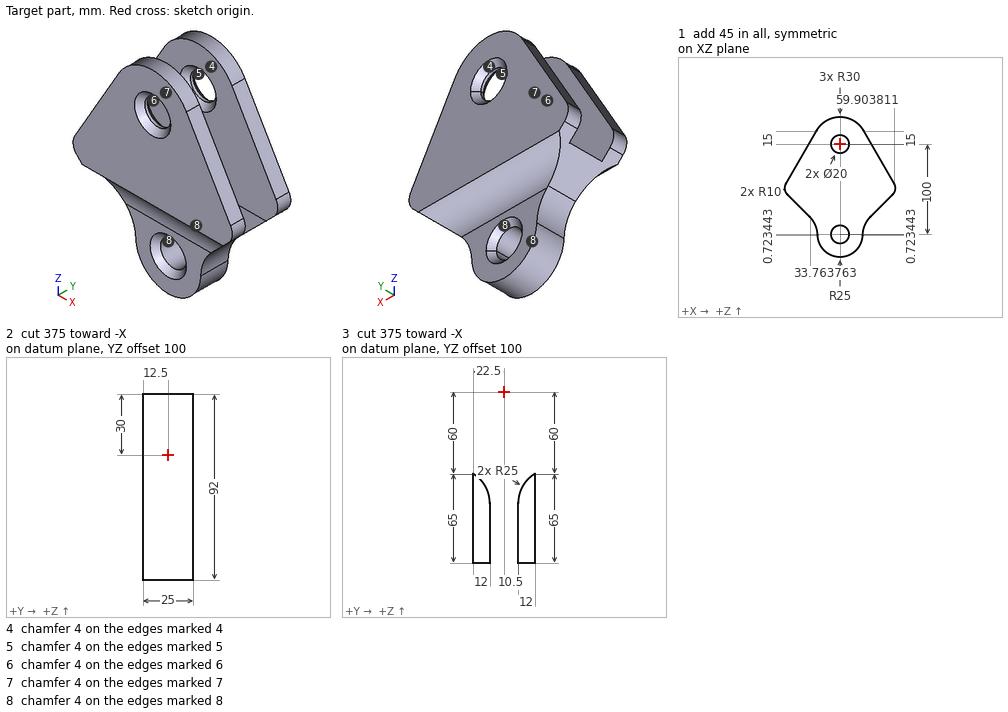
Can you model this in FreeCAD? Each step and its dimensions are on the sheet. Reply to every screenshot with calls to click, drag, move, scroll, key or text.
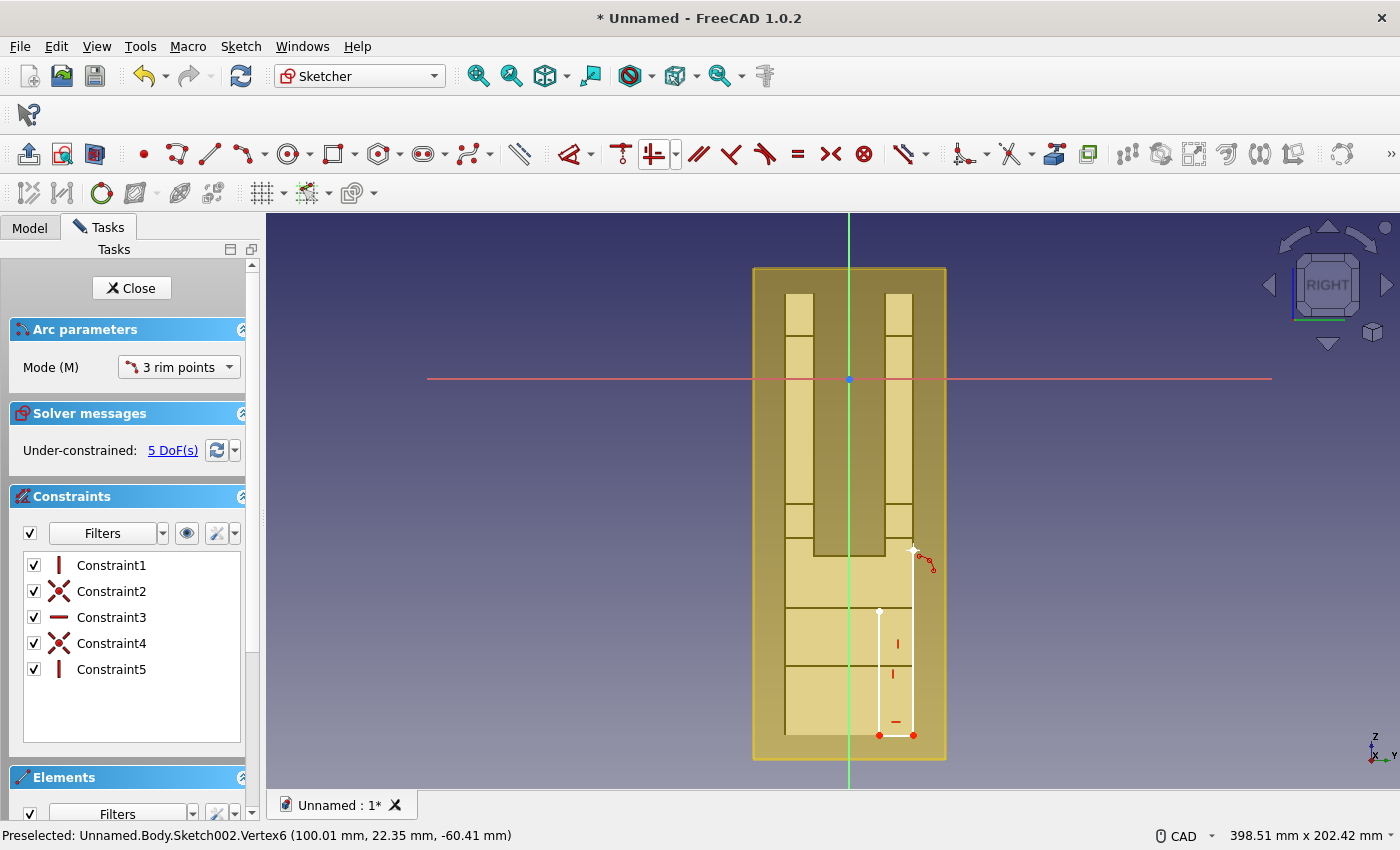
click(913, 551)
click(879, 612)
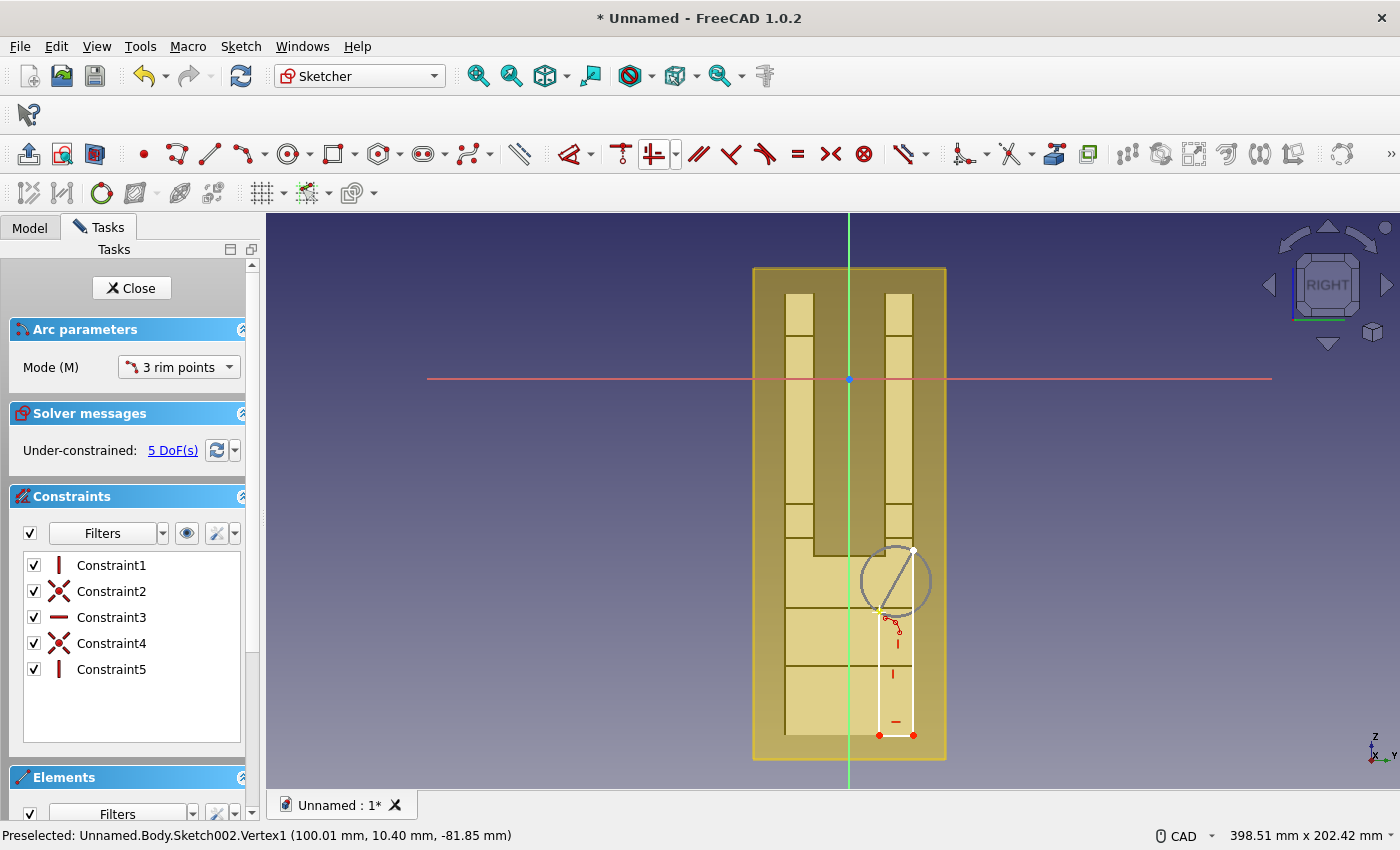
scroll(888, 576, up, 3)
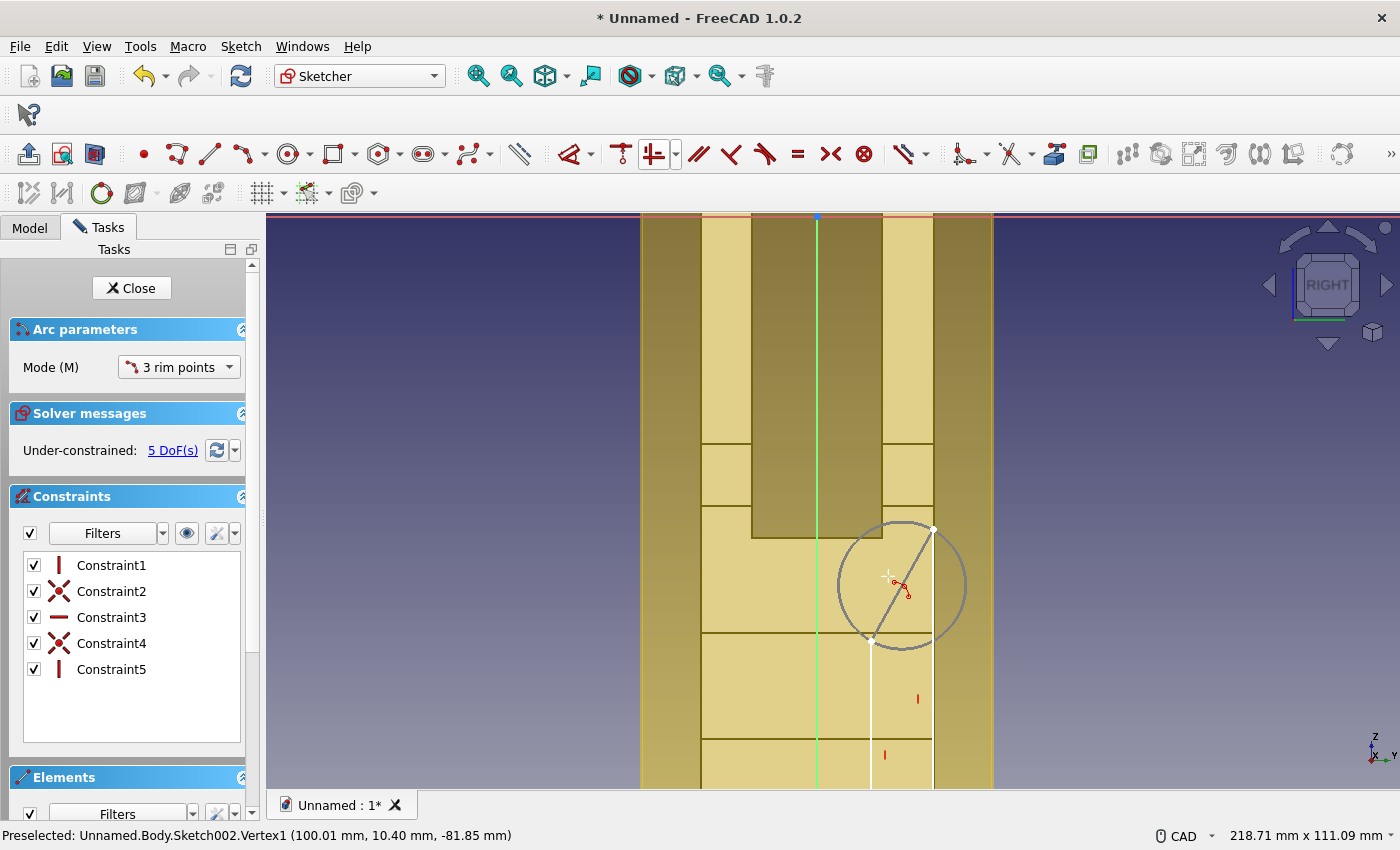
click(888, 575)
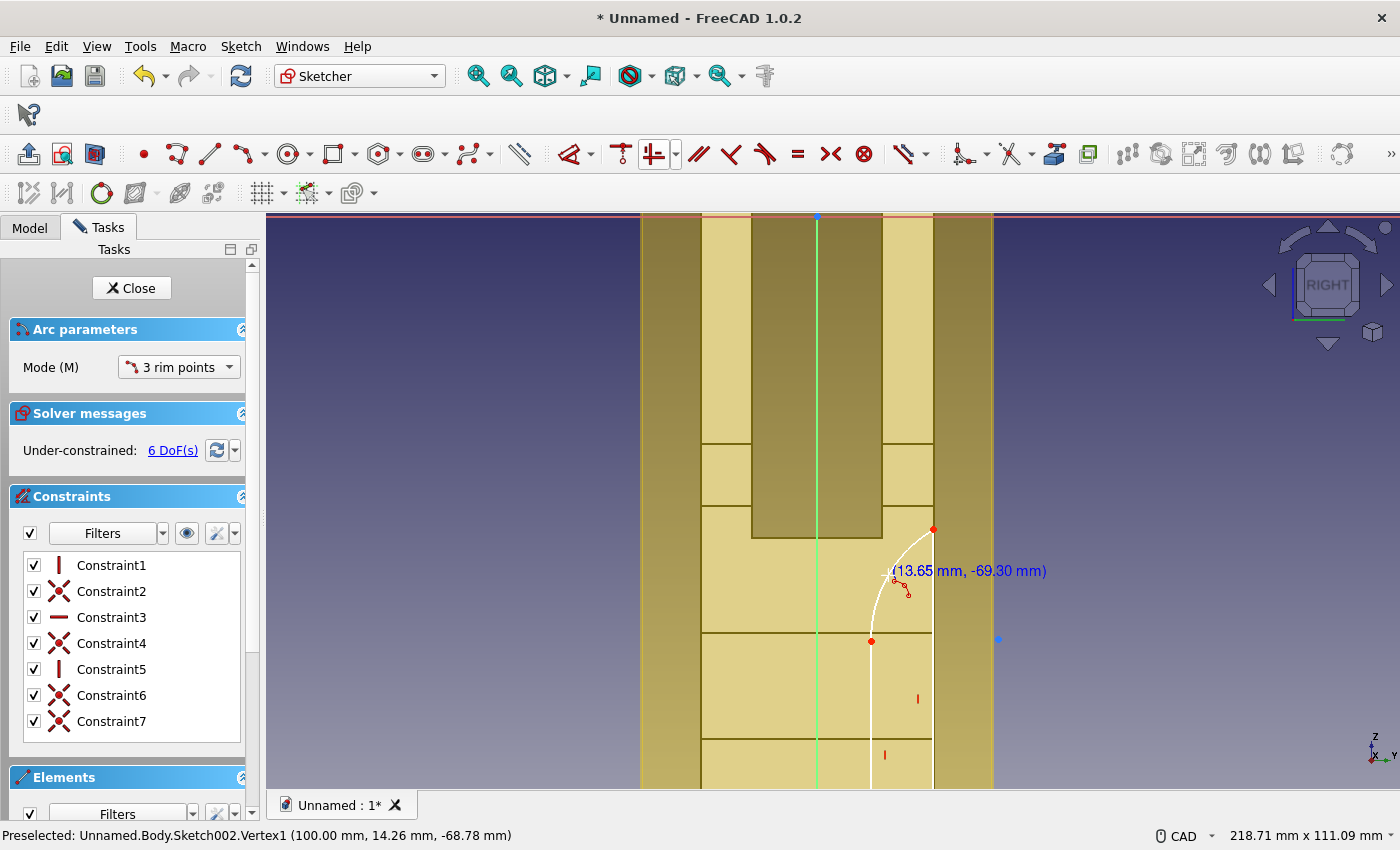
click(177, 154)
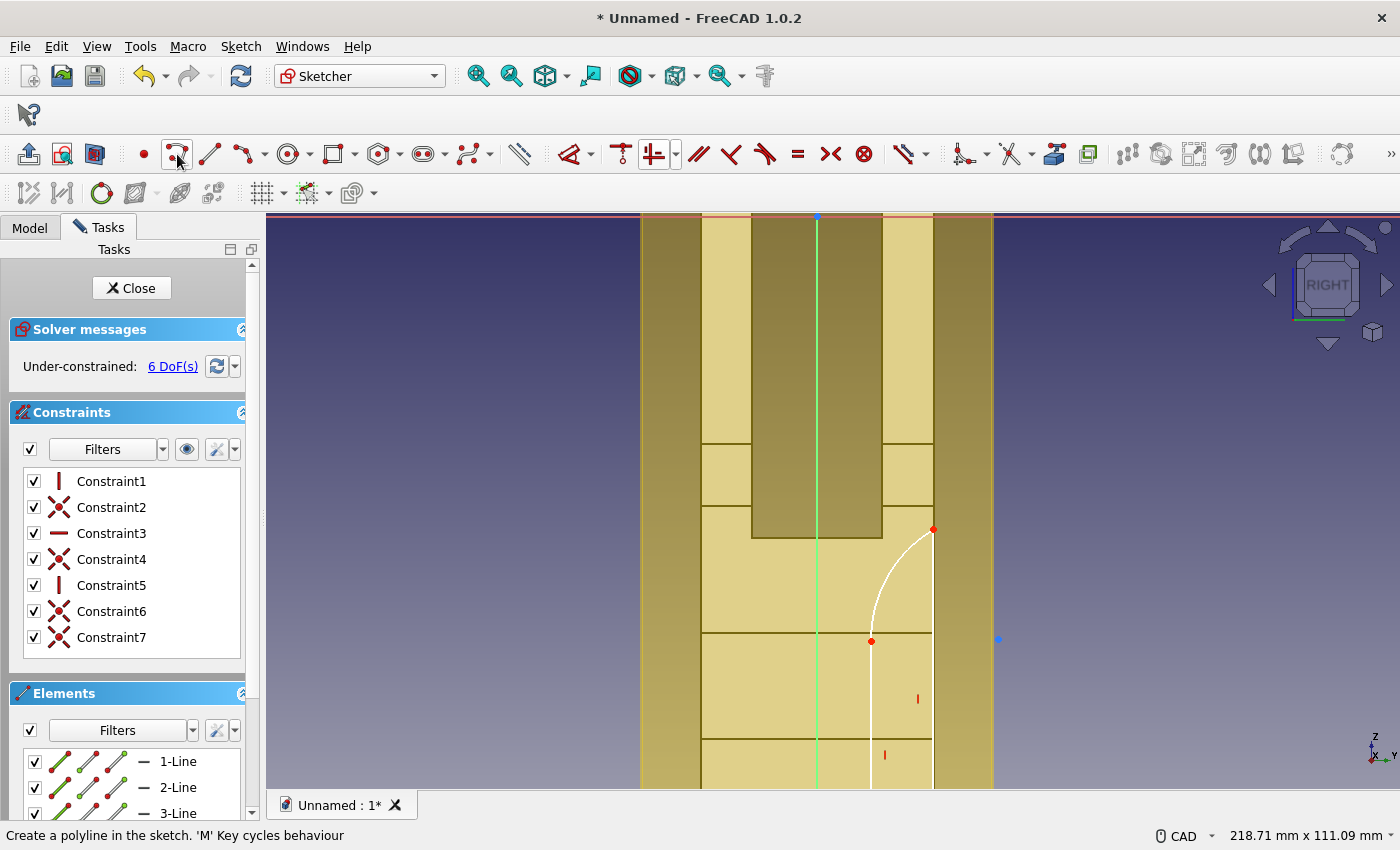
click(701, 528)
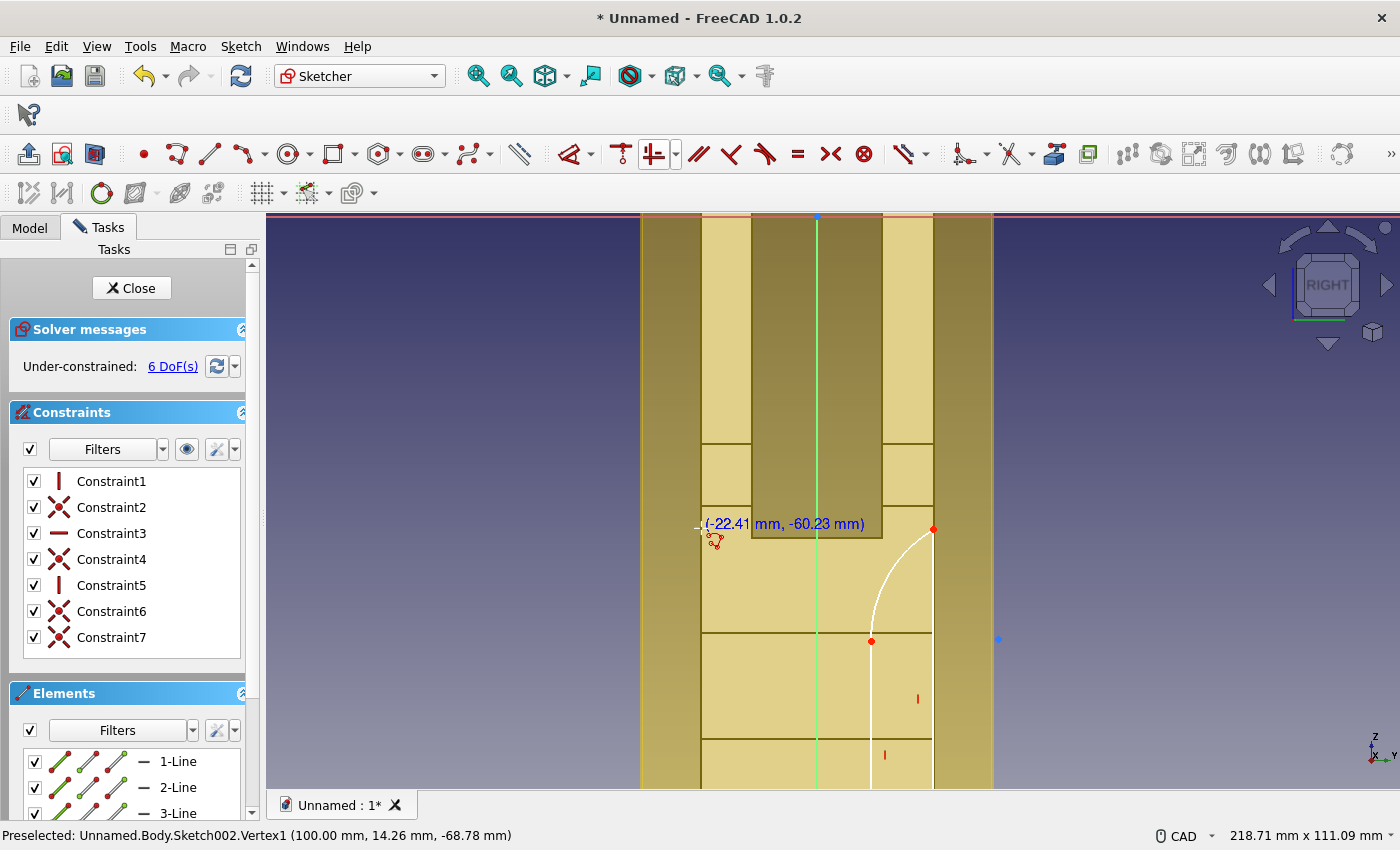
scroll(700, 453, down, 3)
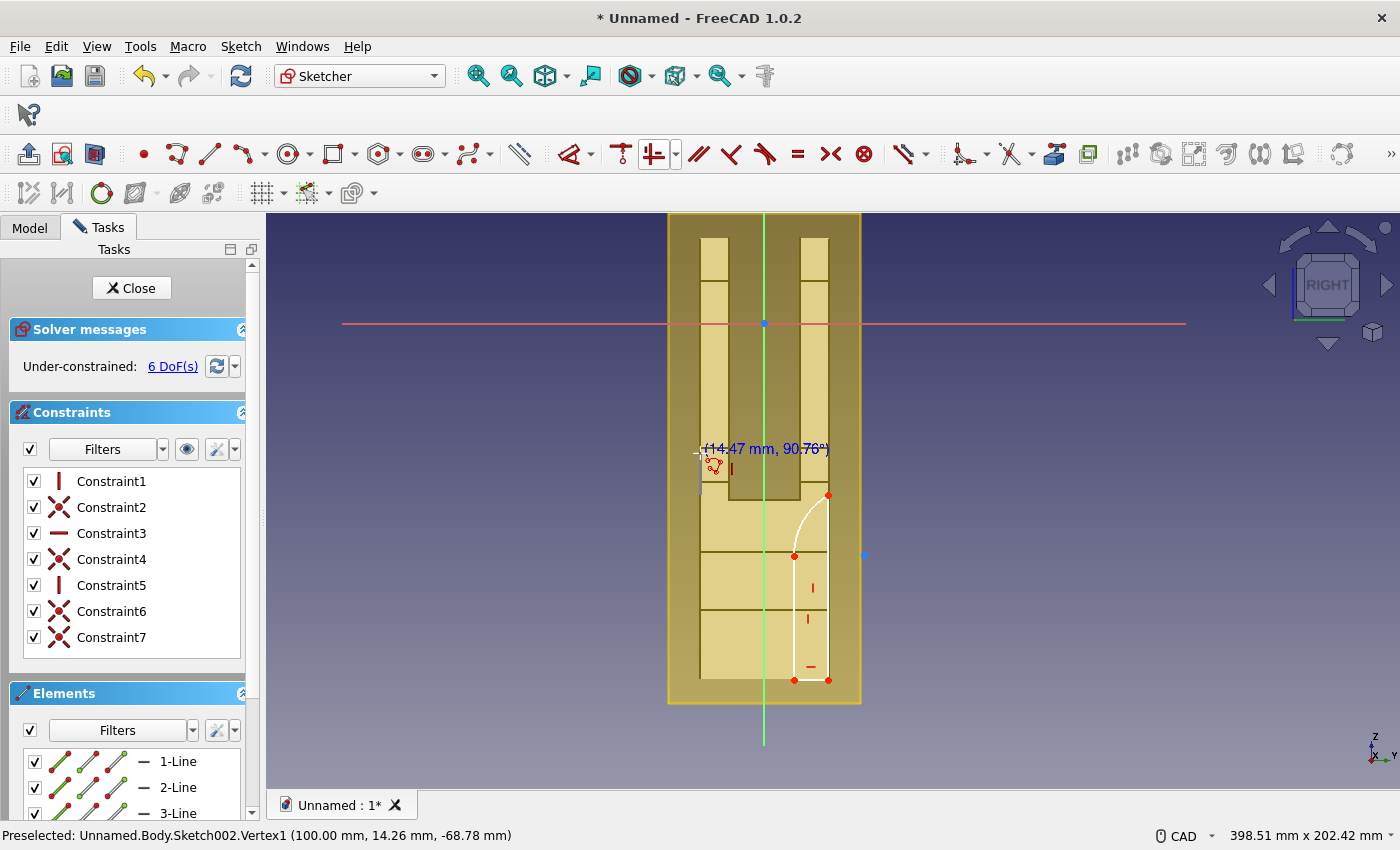
click(701, 679)
click(735, 679)
click(735, 555)
right_click(735, 555)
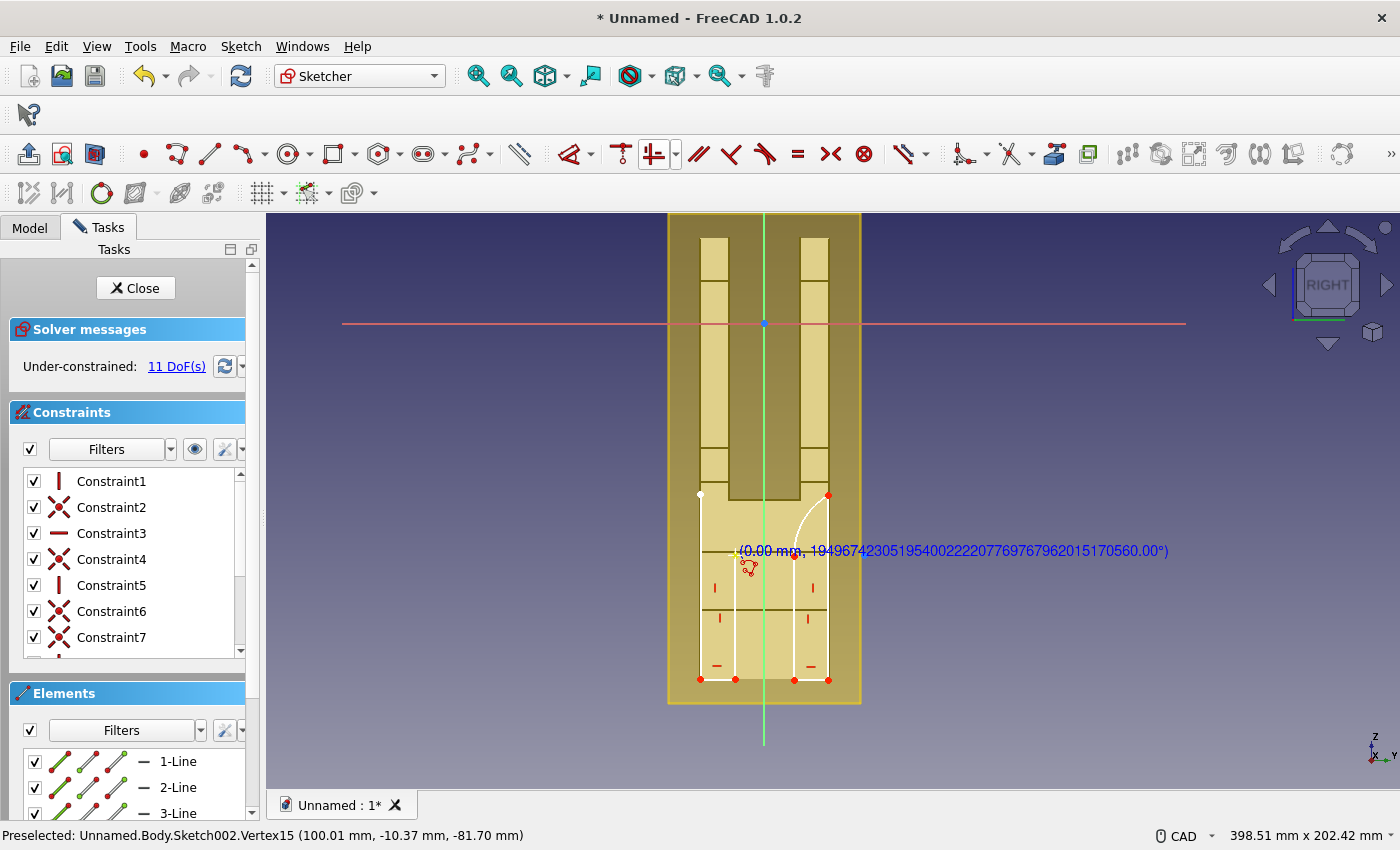
click(242, 154)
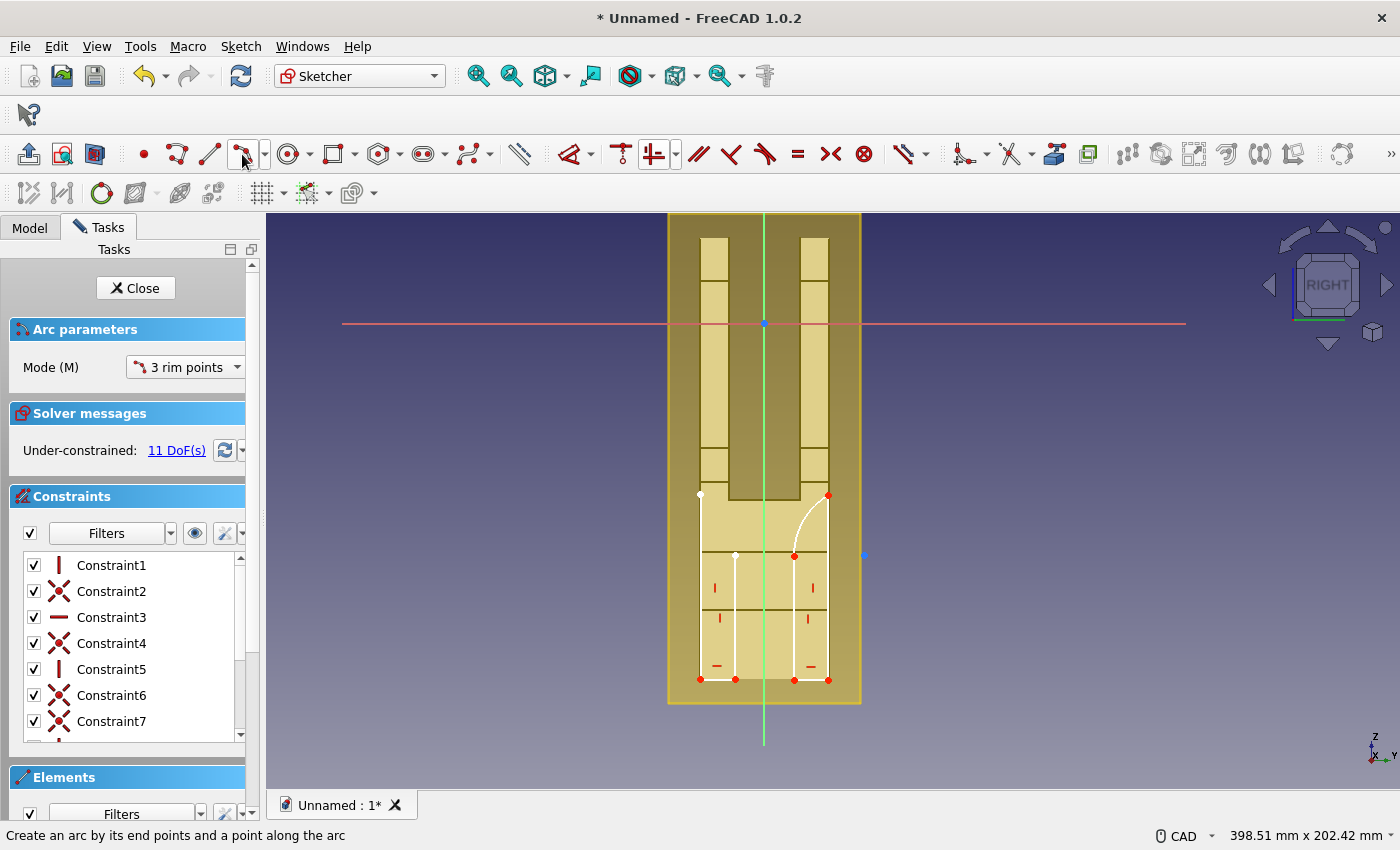
click(735, 556)
click(701, 495)